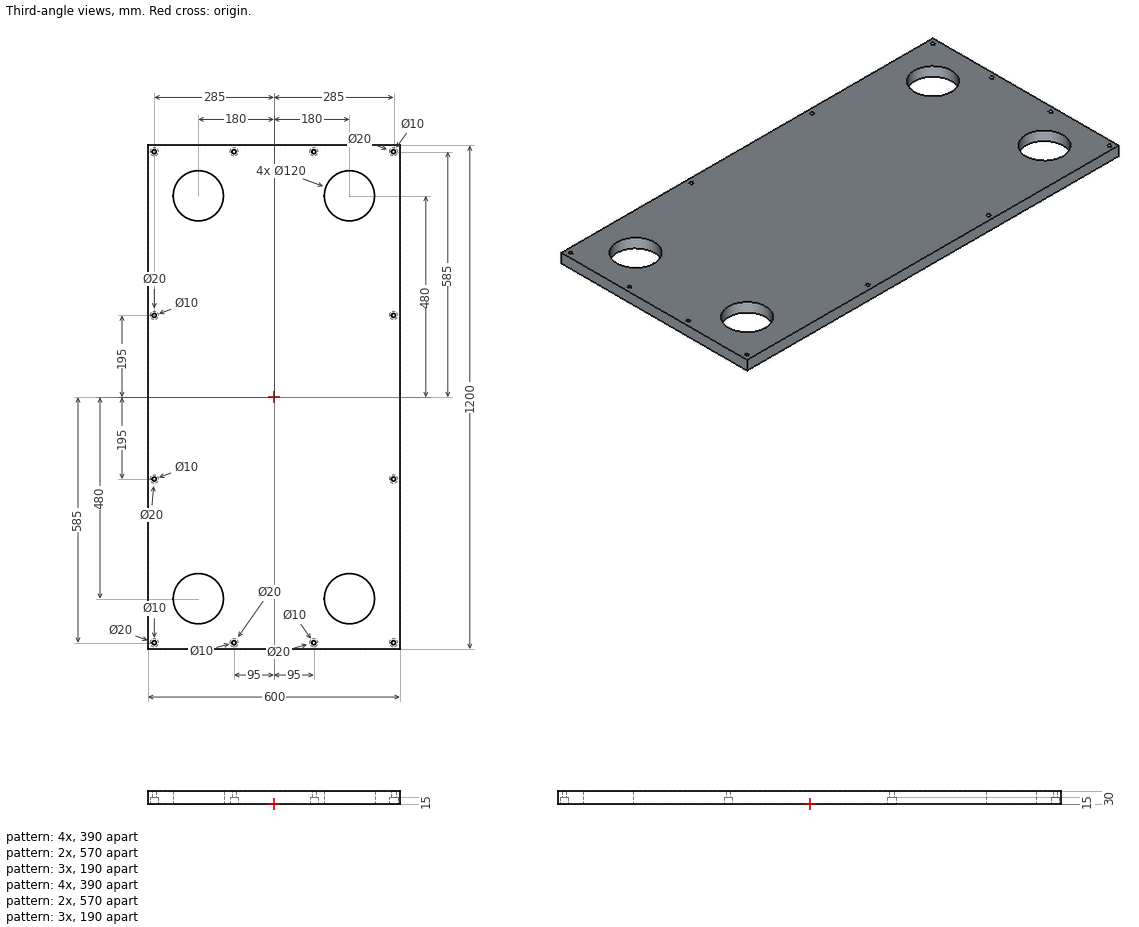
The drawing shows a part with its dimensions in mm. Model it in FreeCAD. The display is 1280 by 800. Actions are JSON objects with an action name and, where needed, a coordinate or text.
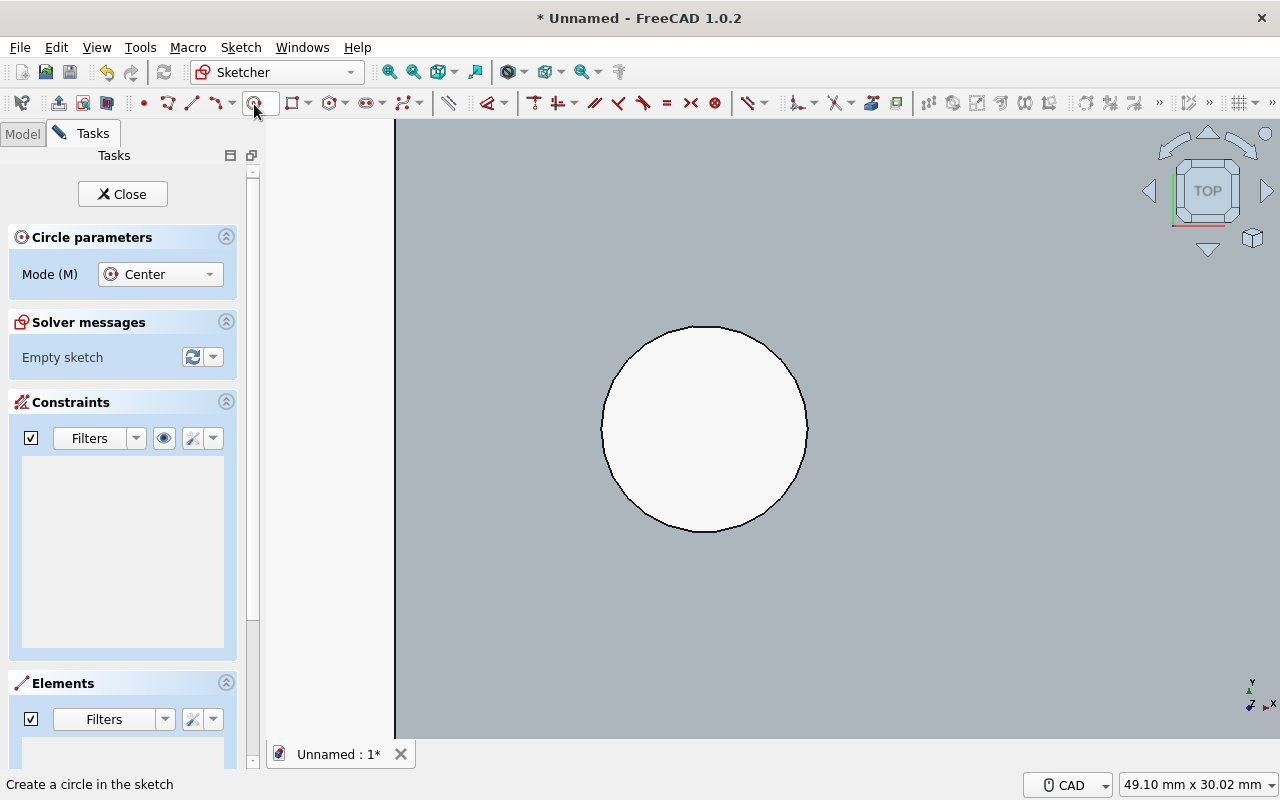
{"action": "left_click", "coordinate": [704, 429]}
{"action": "mouse_move", "coordinate": [851, 283]}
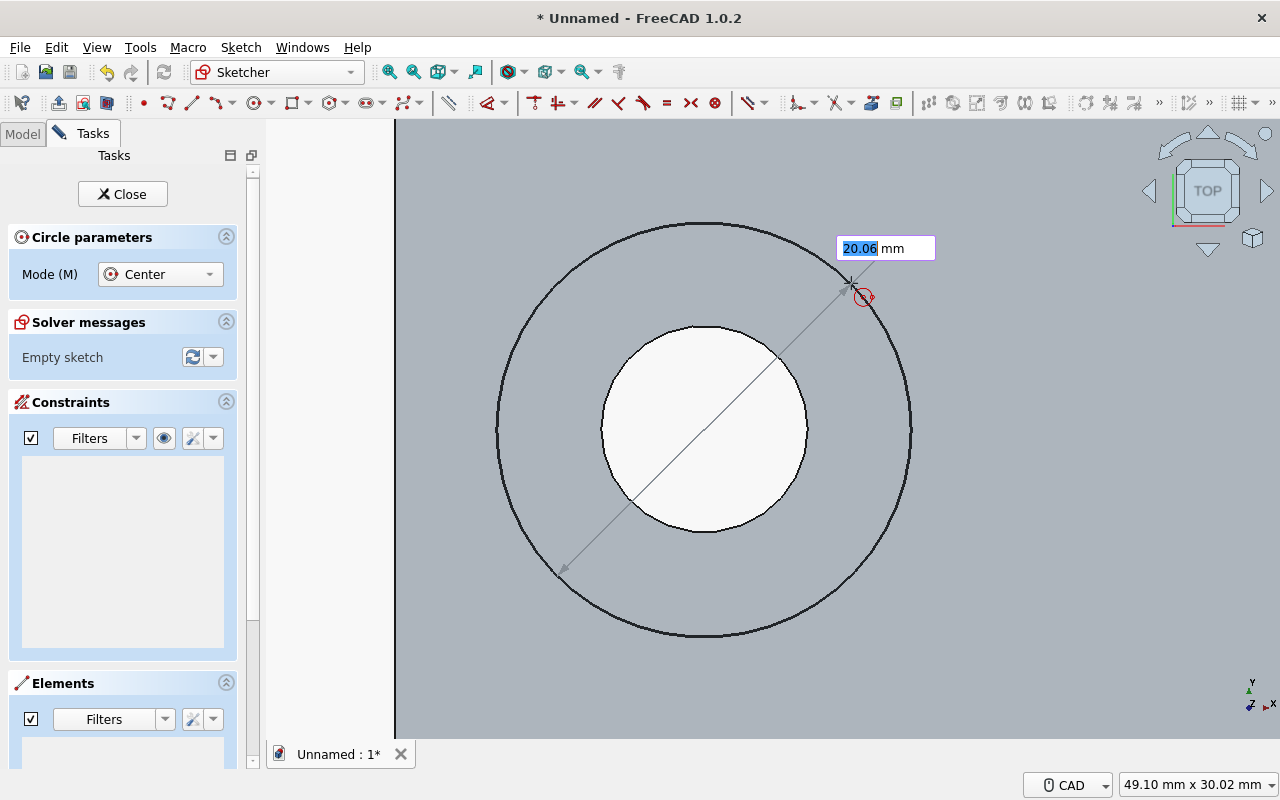
{"action": "type", "text": "20"}
{"action": "key", "text": "Return"}
{"action": "key", "text": "Escape"}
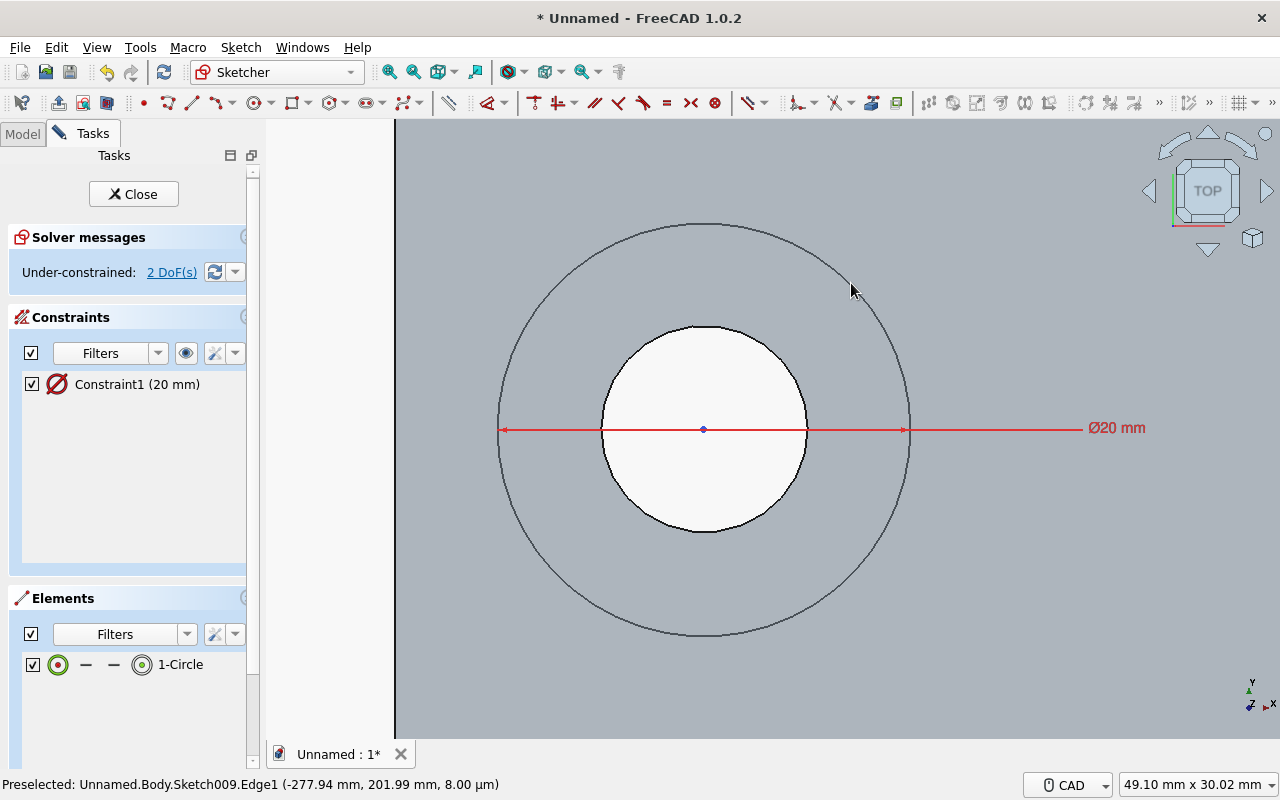
{"action": "left_click", "coordinate": [488, 104]}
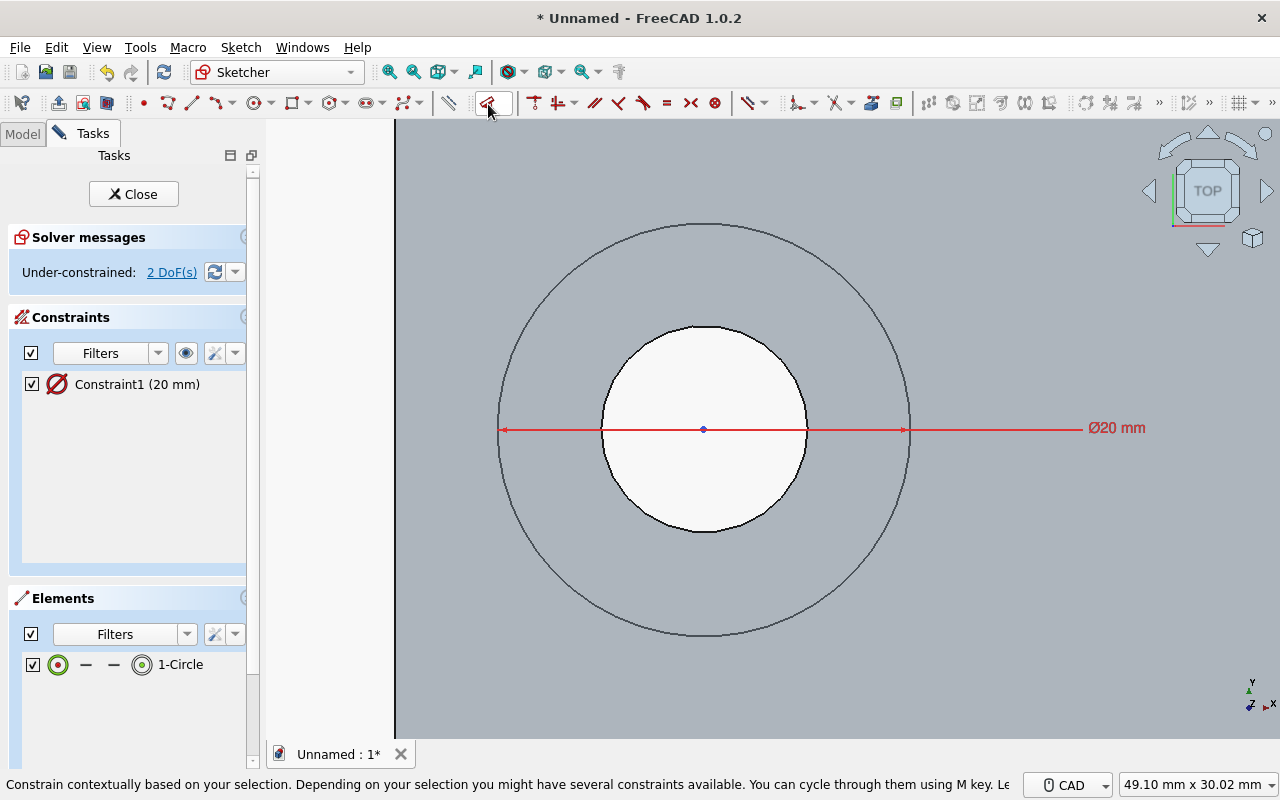
{"action": "left_click", "coordinate": [704, 430]}
{"action": "left_click", "coordinate": [815, 396]}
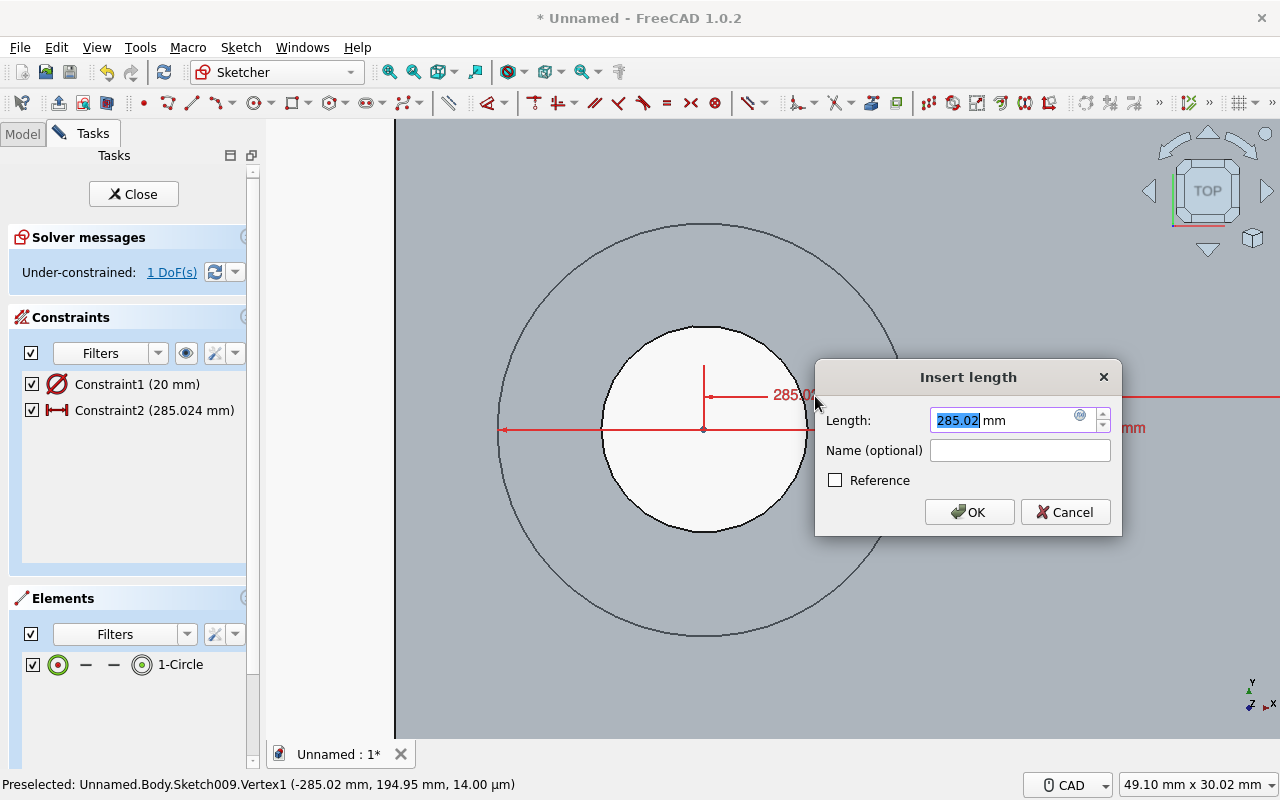
{"action": "type", "text": "285"}
{"action": "key", "text": "Return"}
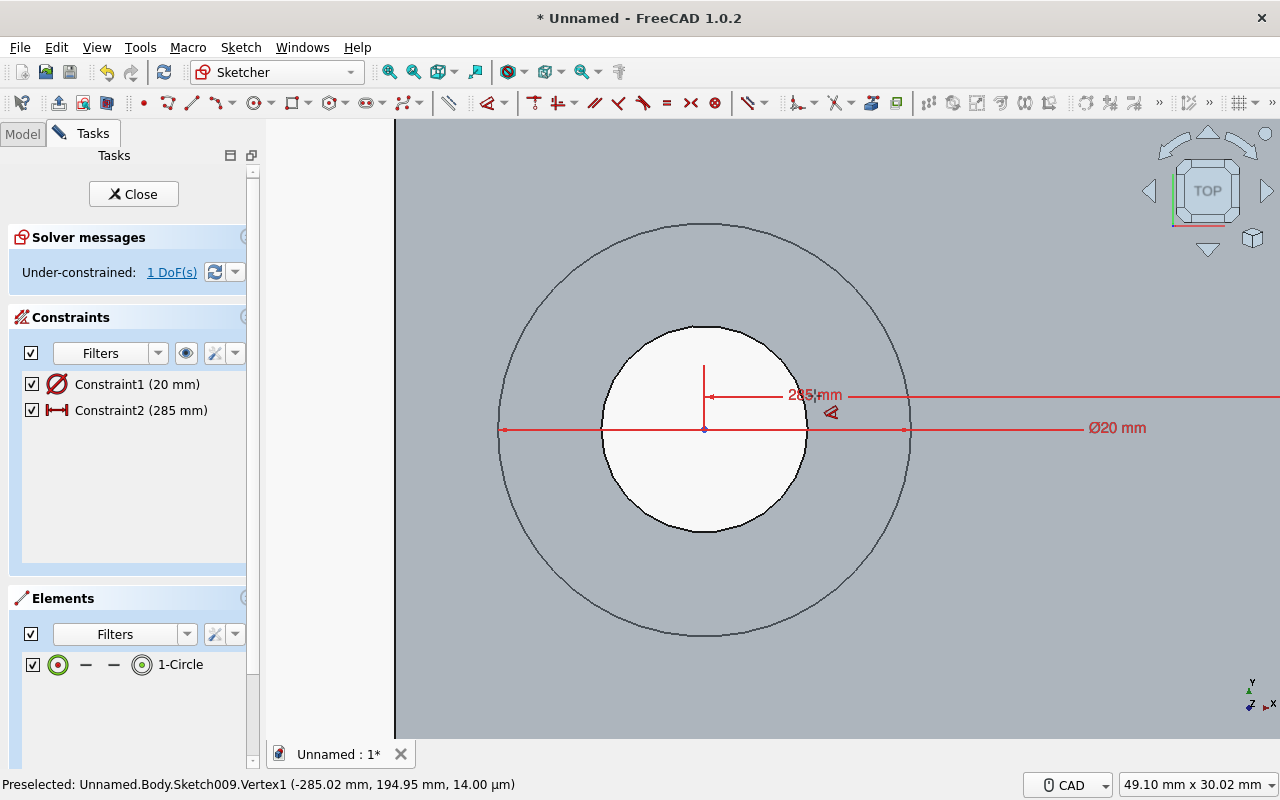
{"action": "left_click", "coordinate": [704, 430]}
{"action": "left_click", "coordinate": [670, 570]}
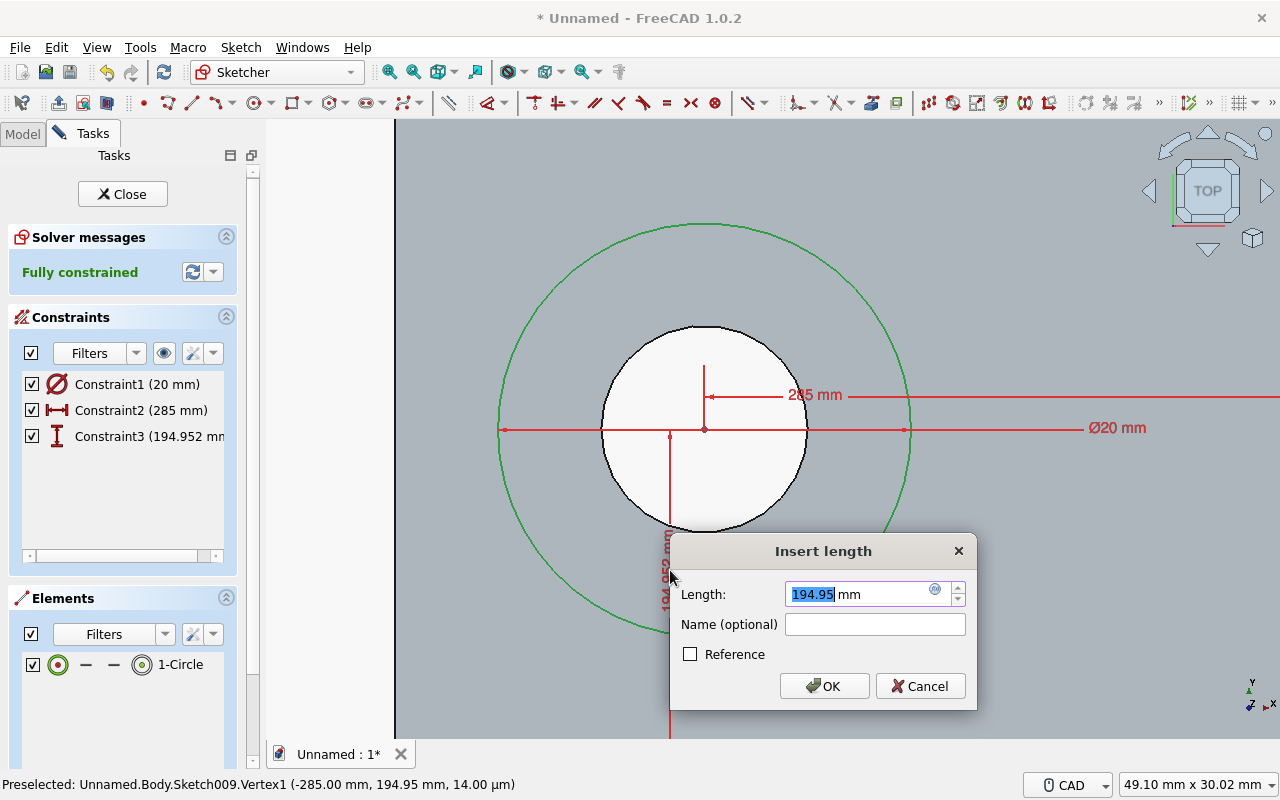
{"action": "type", "text": "195"}
{"action": "key", "text": "Return"}
{"action": "key", "text": "Escape"}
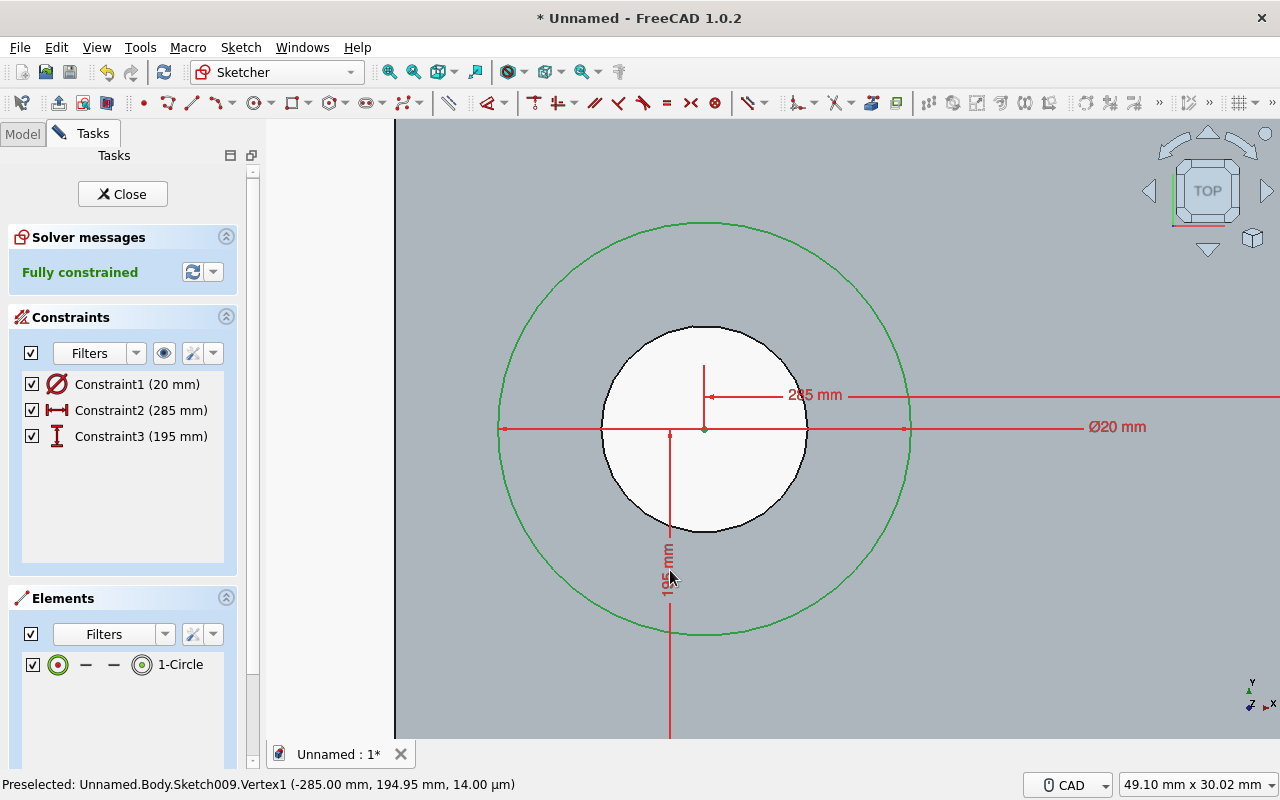
{"action": "left_click", "coordinate": [123, 194]}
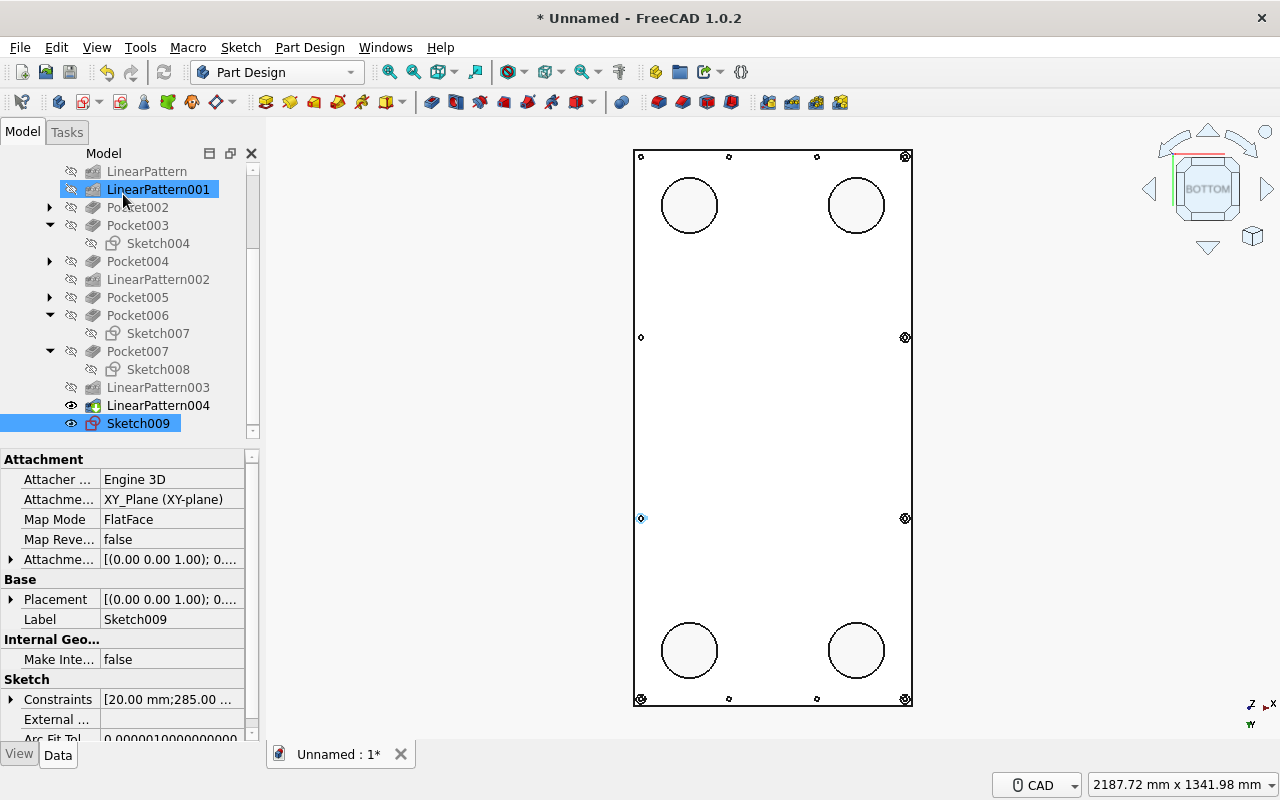
{"action": "left_click", "coordinate": [432, 102]}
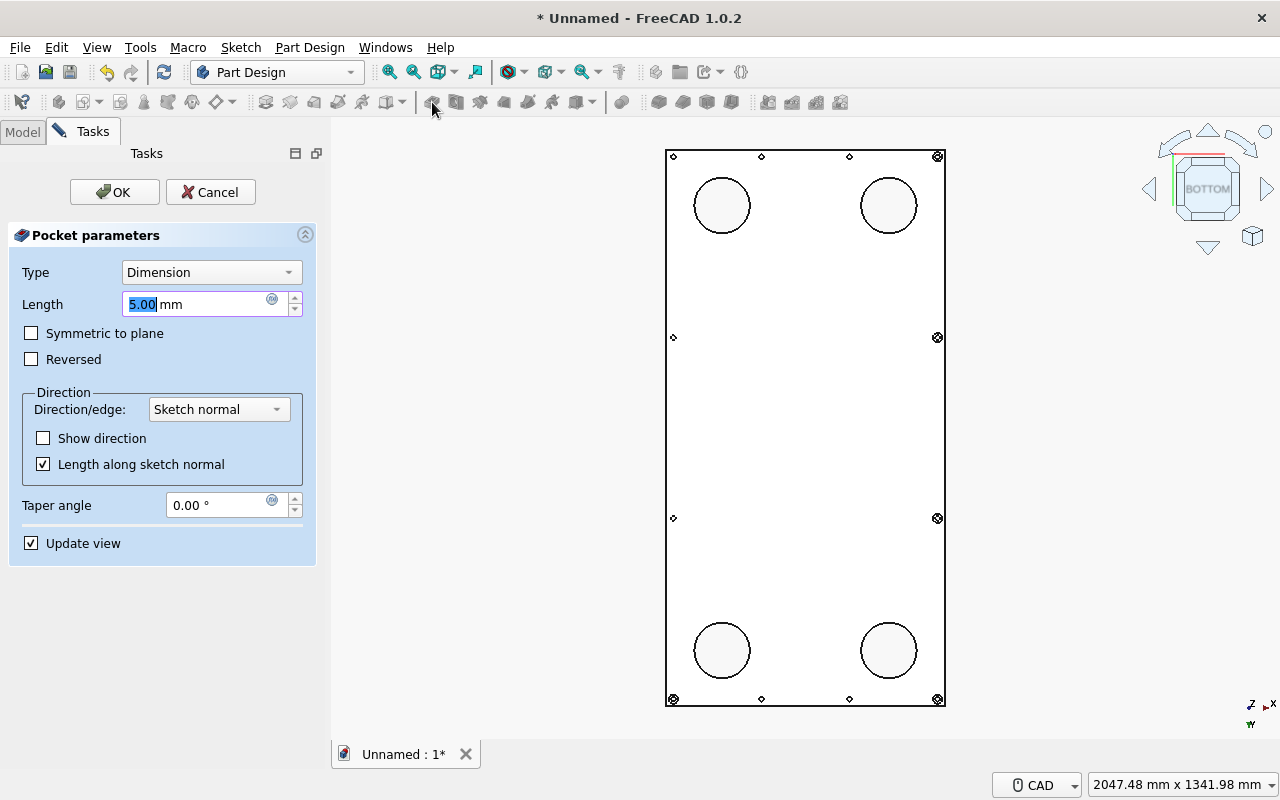
{"action": "type", "text": "15"}
{"action": "key", "text": "Tab"}